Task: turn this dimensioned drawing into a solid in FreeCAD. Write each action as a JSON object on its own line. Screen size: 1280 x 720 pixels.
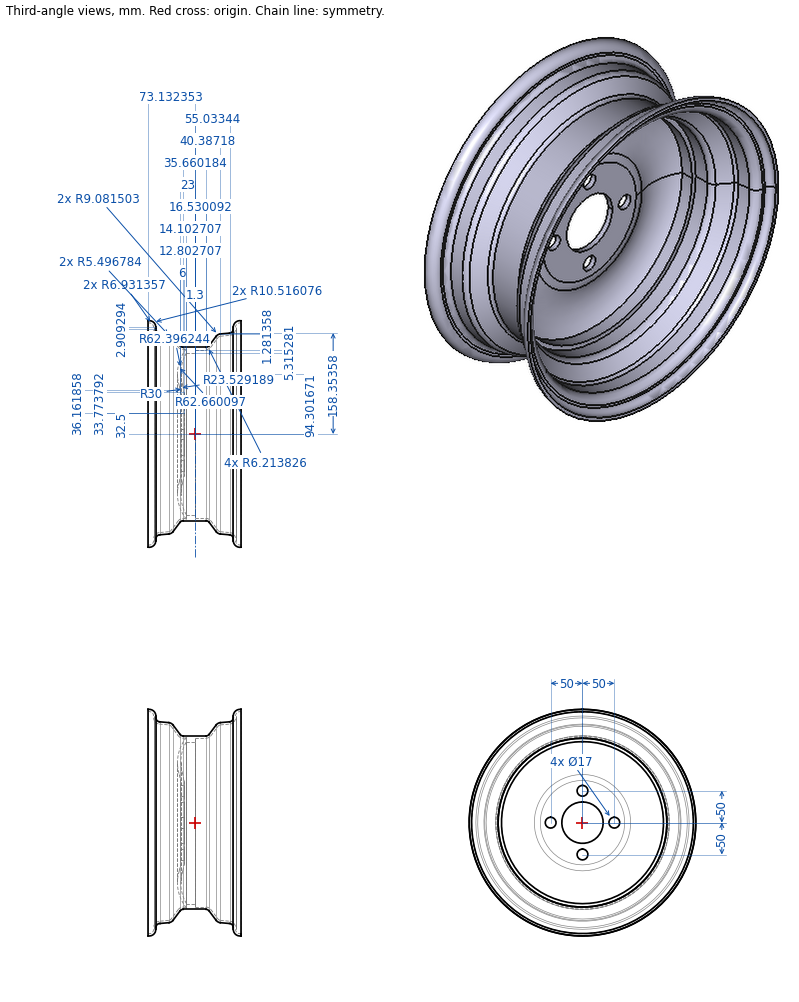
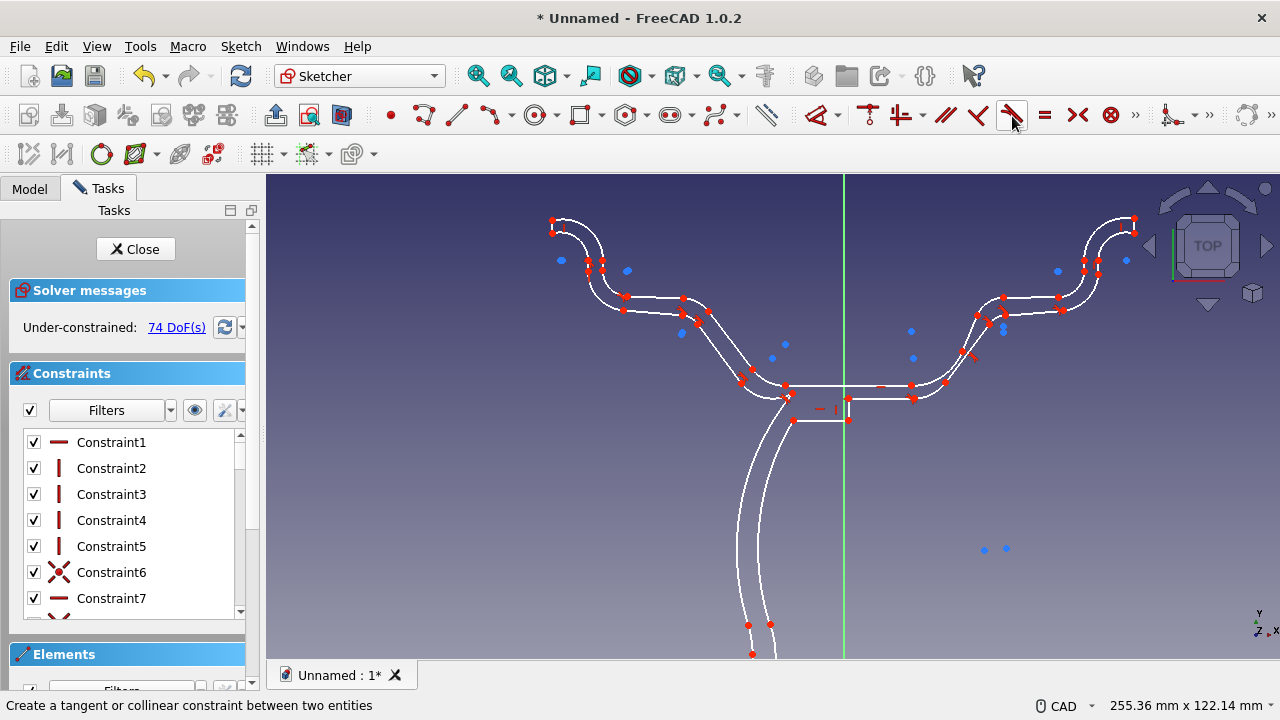
{"action": "left_click", "coordinate": [641, 312]}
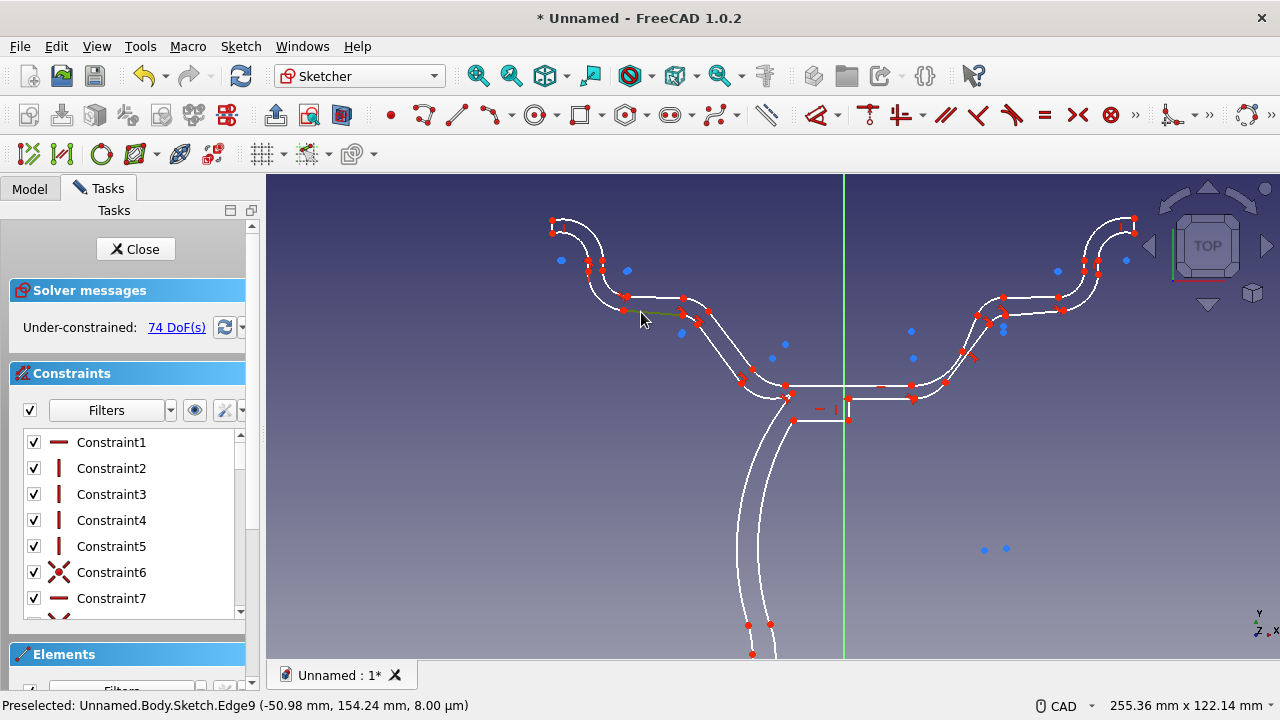
{"action": "scroll", "coordinate": [691, 318], "scroll_direction": "up", "scroll_amount": 3}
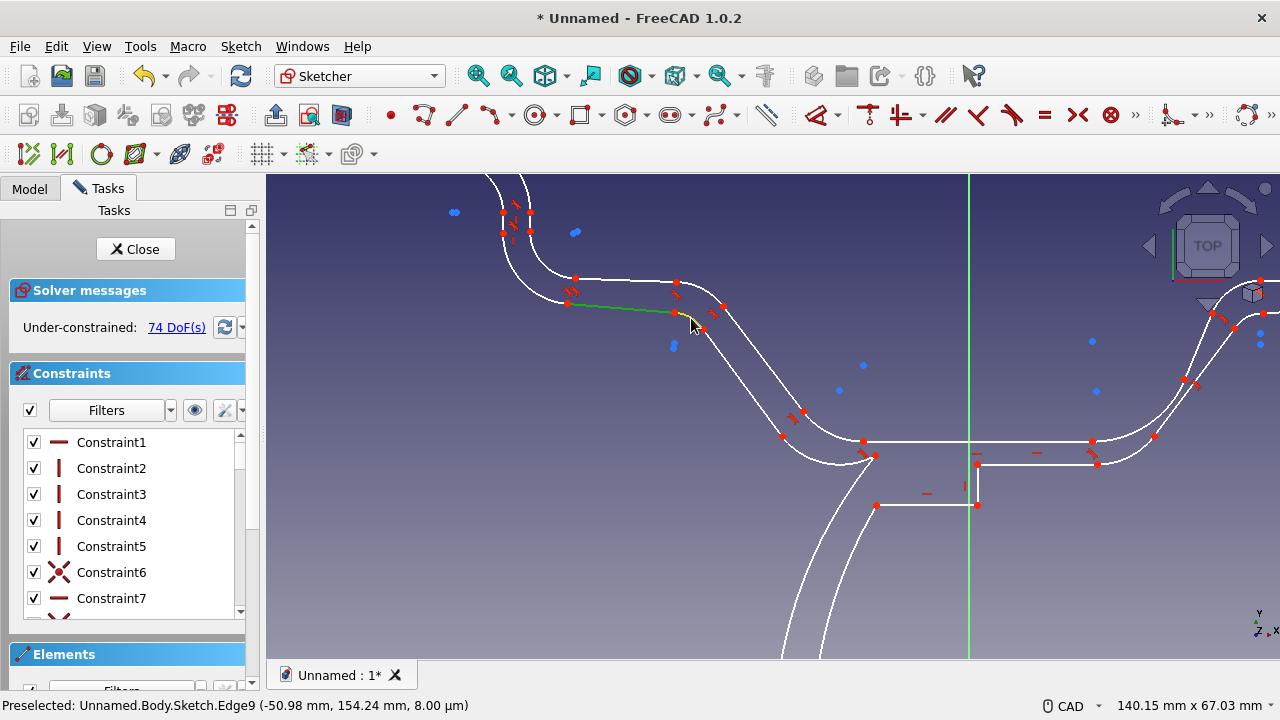
{"action": "left_click", "coordinate": [691, 318]}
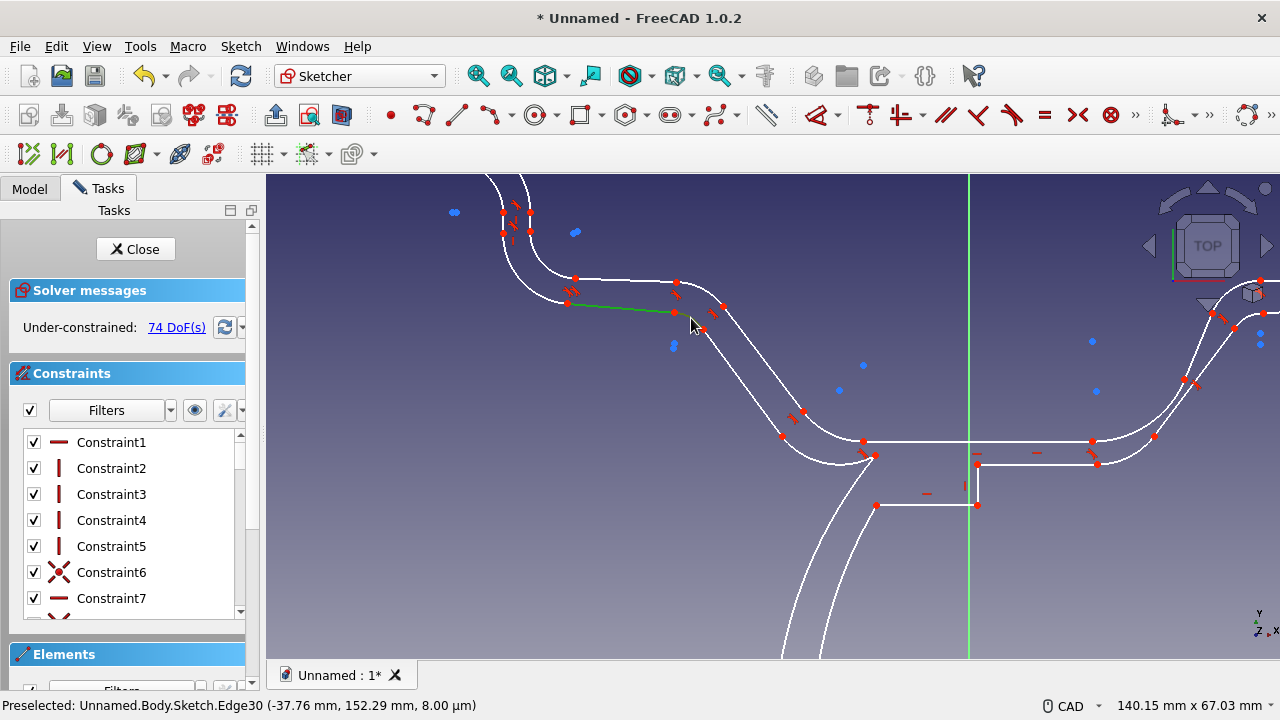
{"action": "key", "text": "t"}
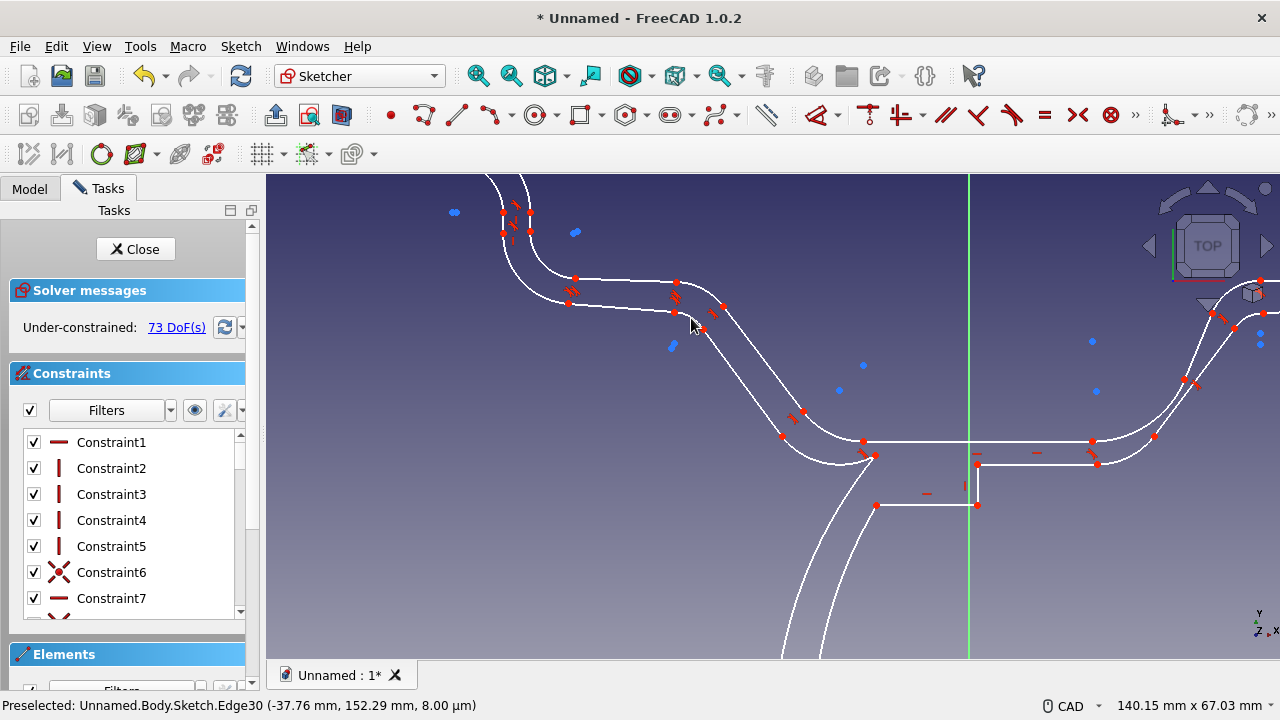
{"action": "left_click", "coordinate": [727, 362]}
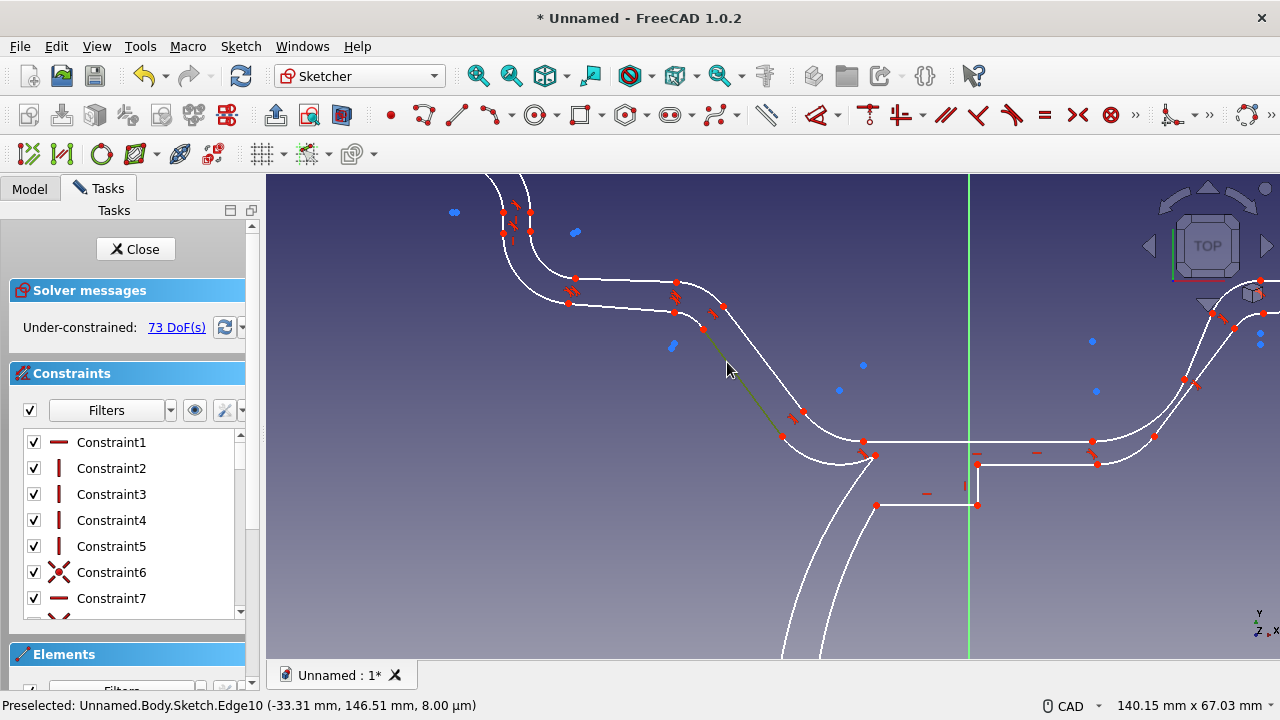
{"action": "scroll", "coordinate": [697, 321], "scroll_direction": "up", "scroll_amount": 2}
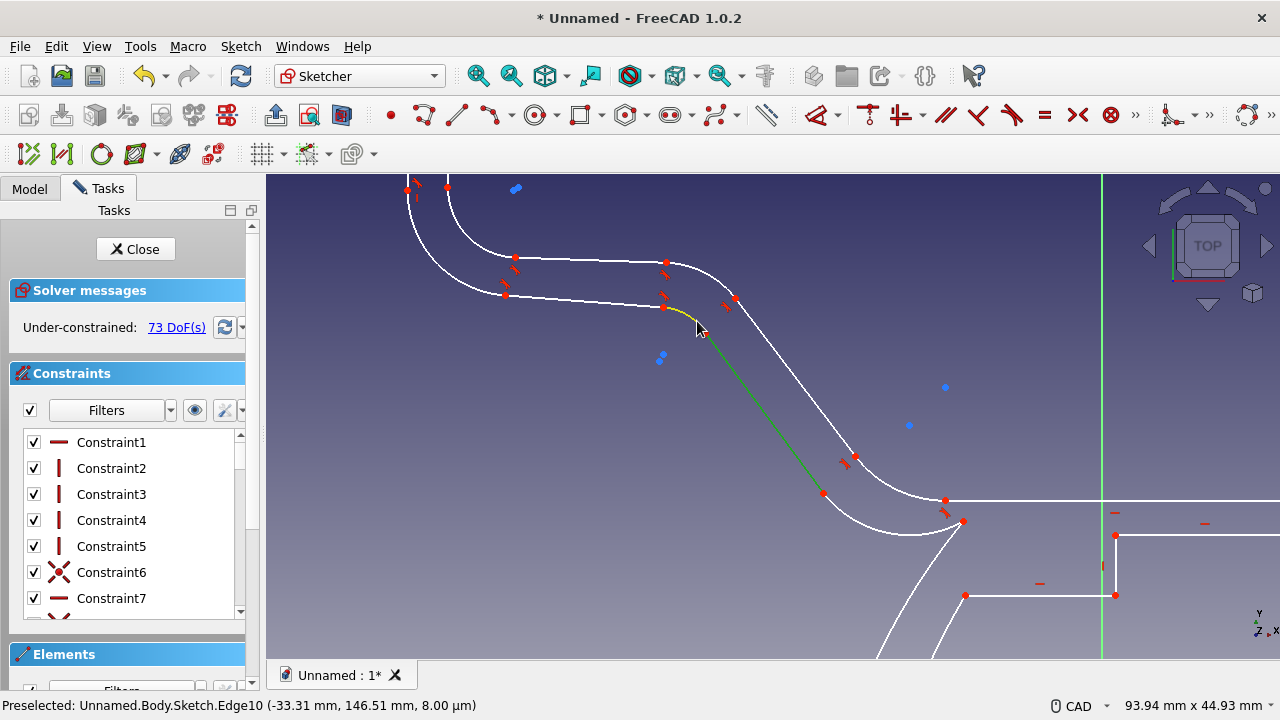
{"action": "left_click", "coordinate": [696, 321]}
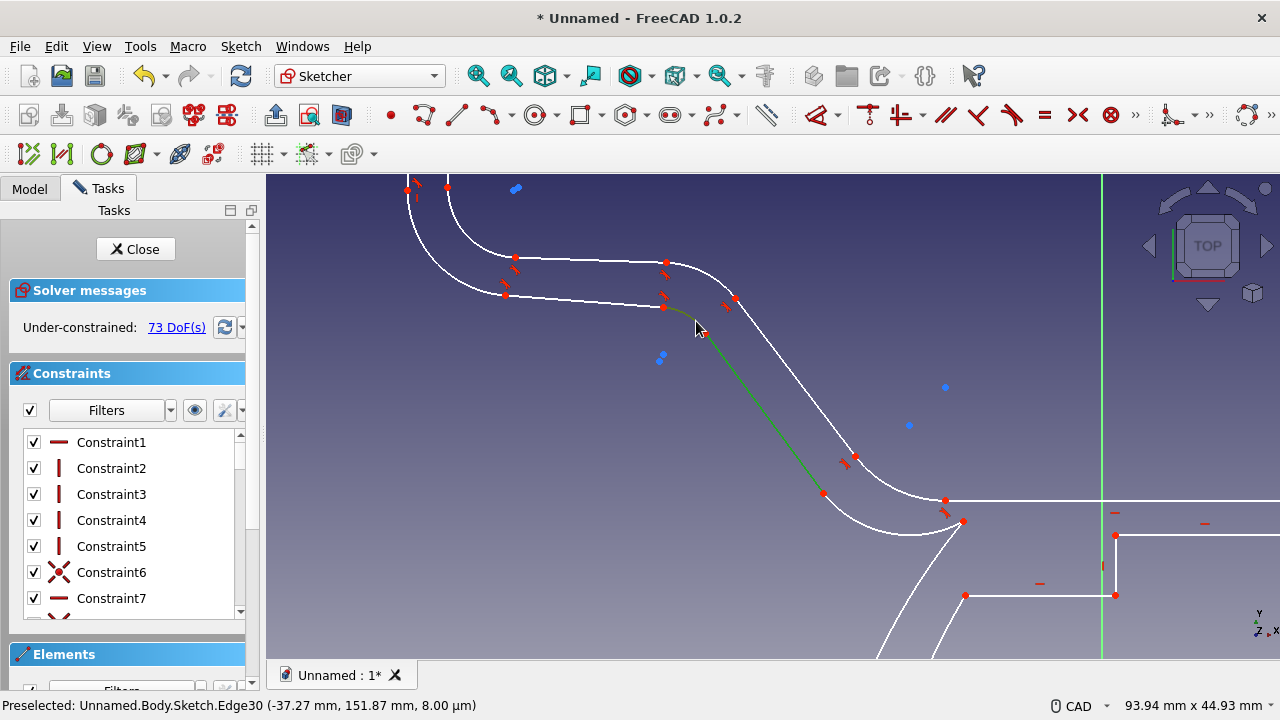
{"action": "key", "text": "t"}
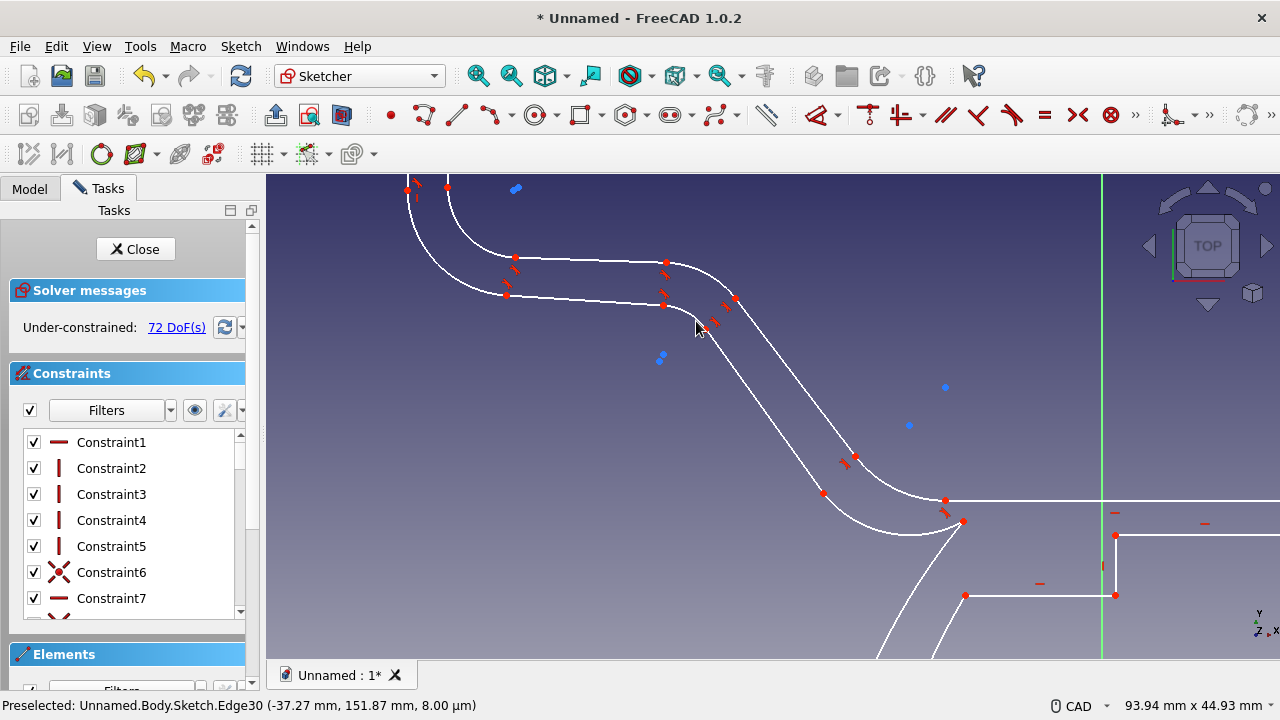
{"action": "scroll", "coordinate": [626, 300], "scroll_direction": "down", "scroll_amount": 9}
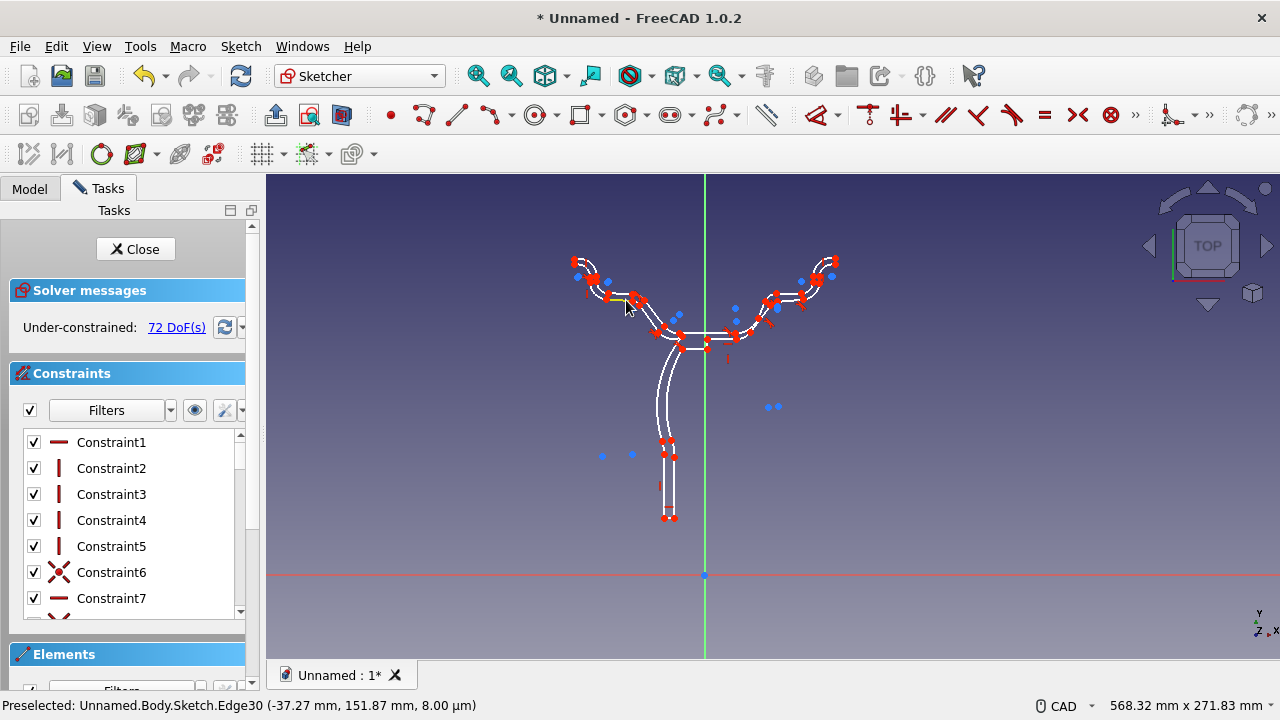
{"action": "scroll", "coordinate": [645, 313], "scroll_direction": "up", "scroll_amount": 4}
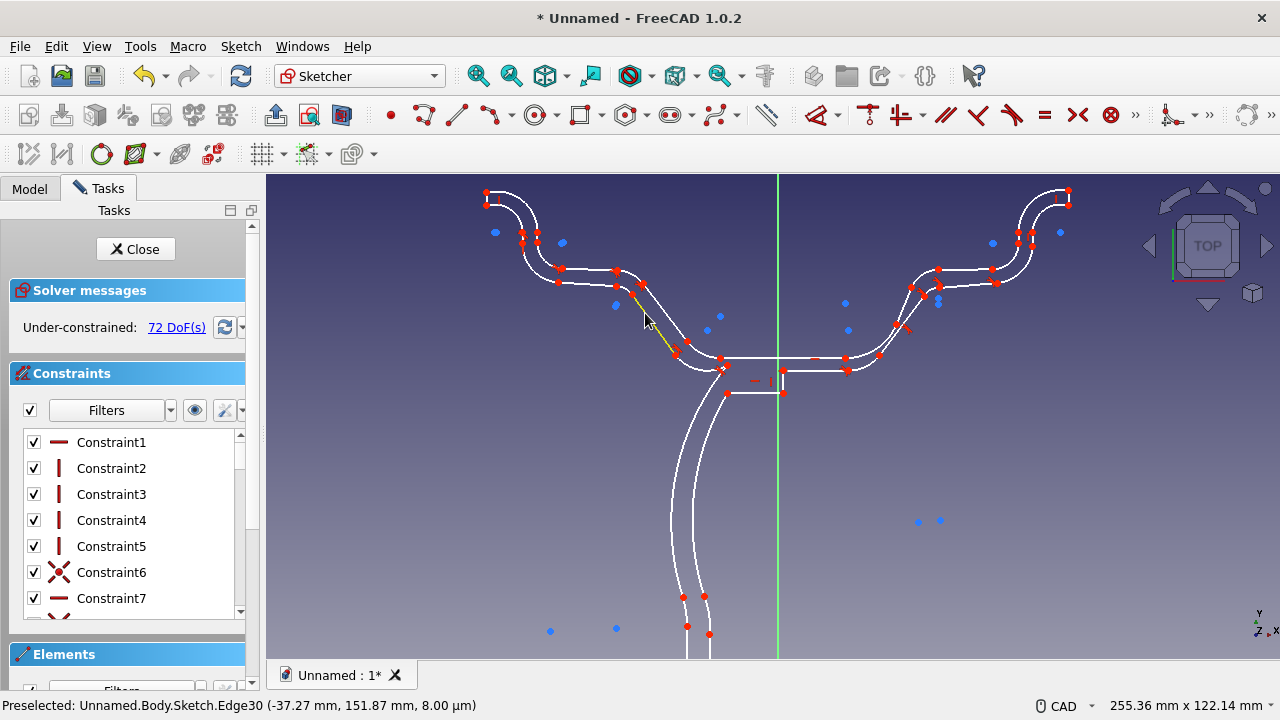
{"action": "left_click", "coordinate": [645, 313]}